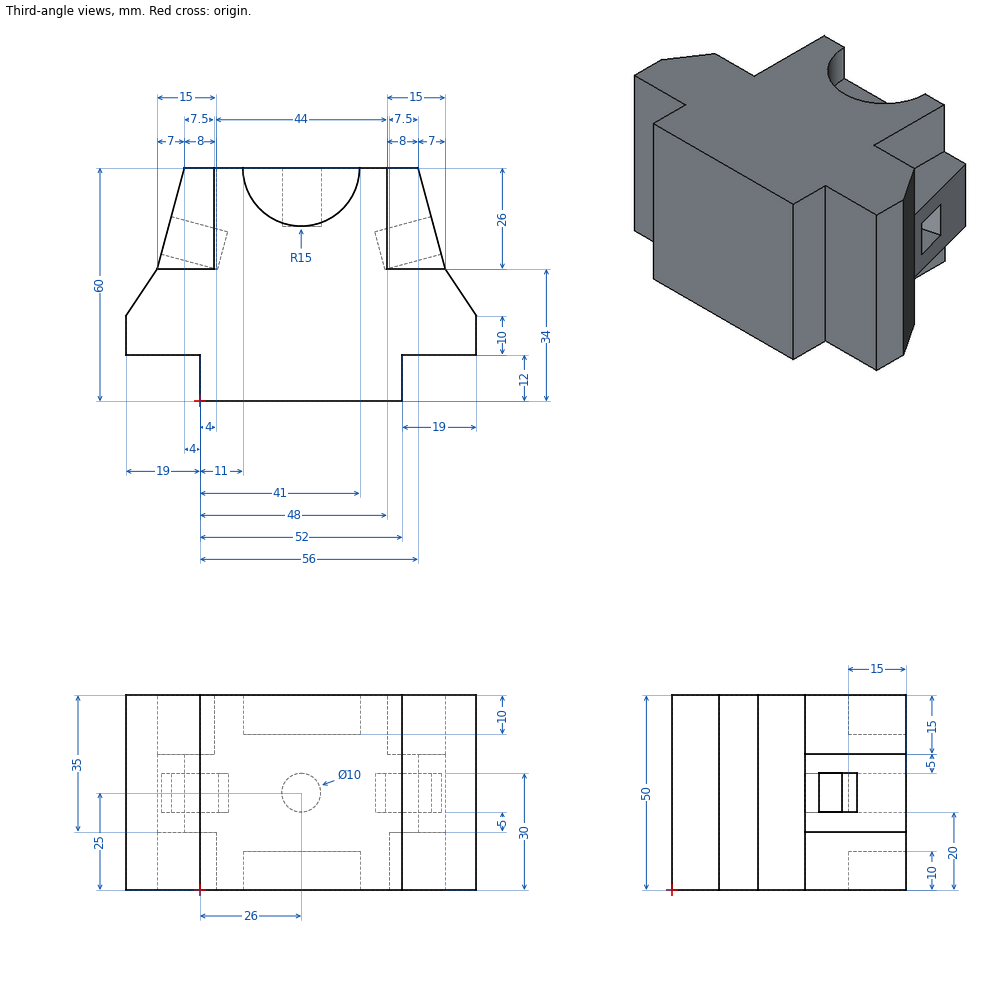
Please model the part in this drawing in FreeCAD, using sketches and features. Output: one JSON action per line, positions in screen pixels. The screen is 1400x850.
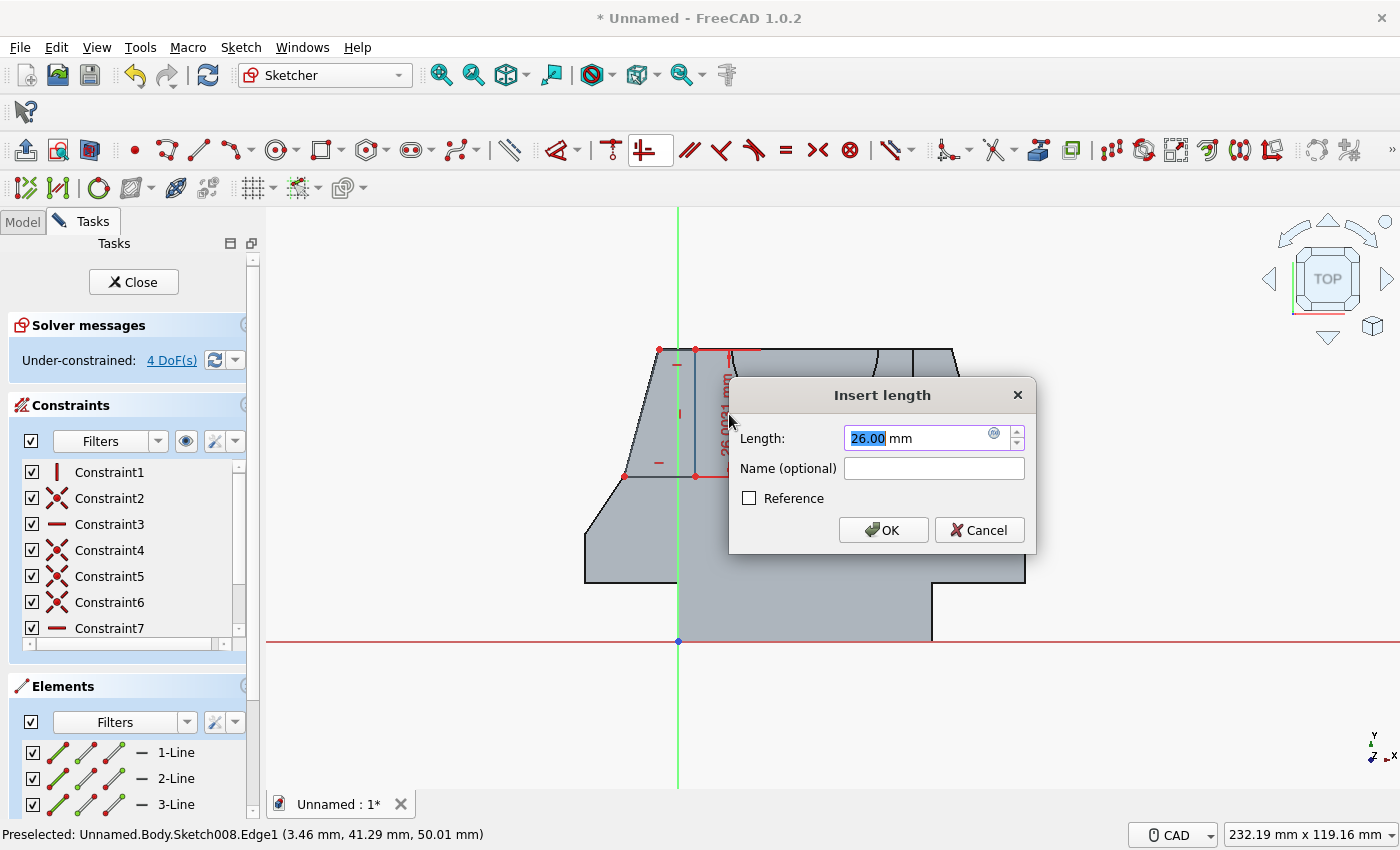
{"action": "type", "text": "26"}
{"action": "key", "text": "Return"}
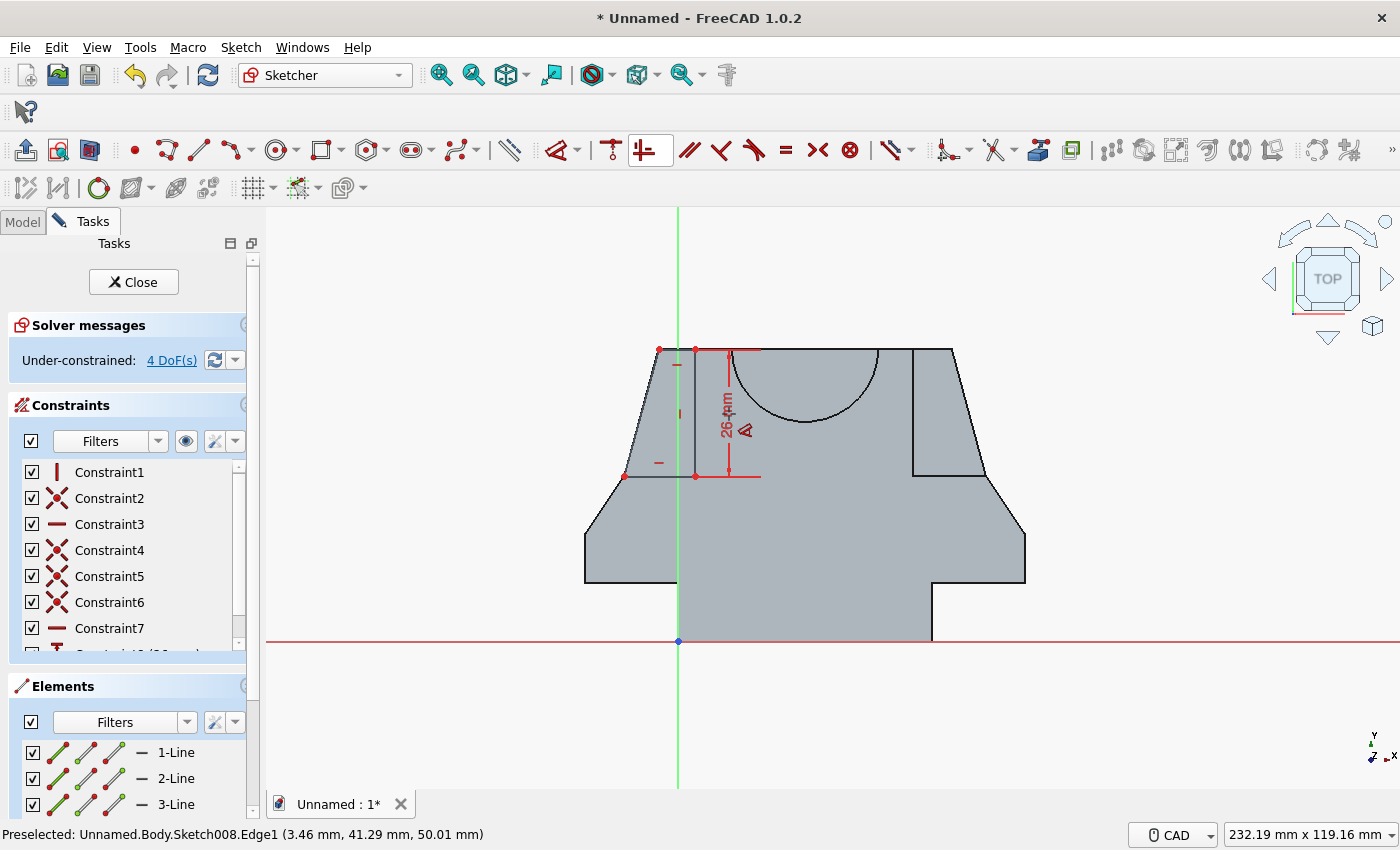
{"action": "scroll", "coordinate": [659, 350], "scroll_direction": "up", "scroll_amount": 4}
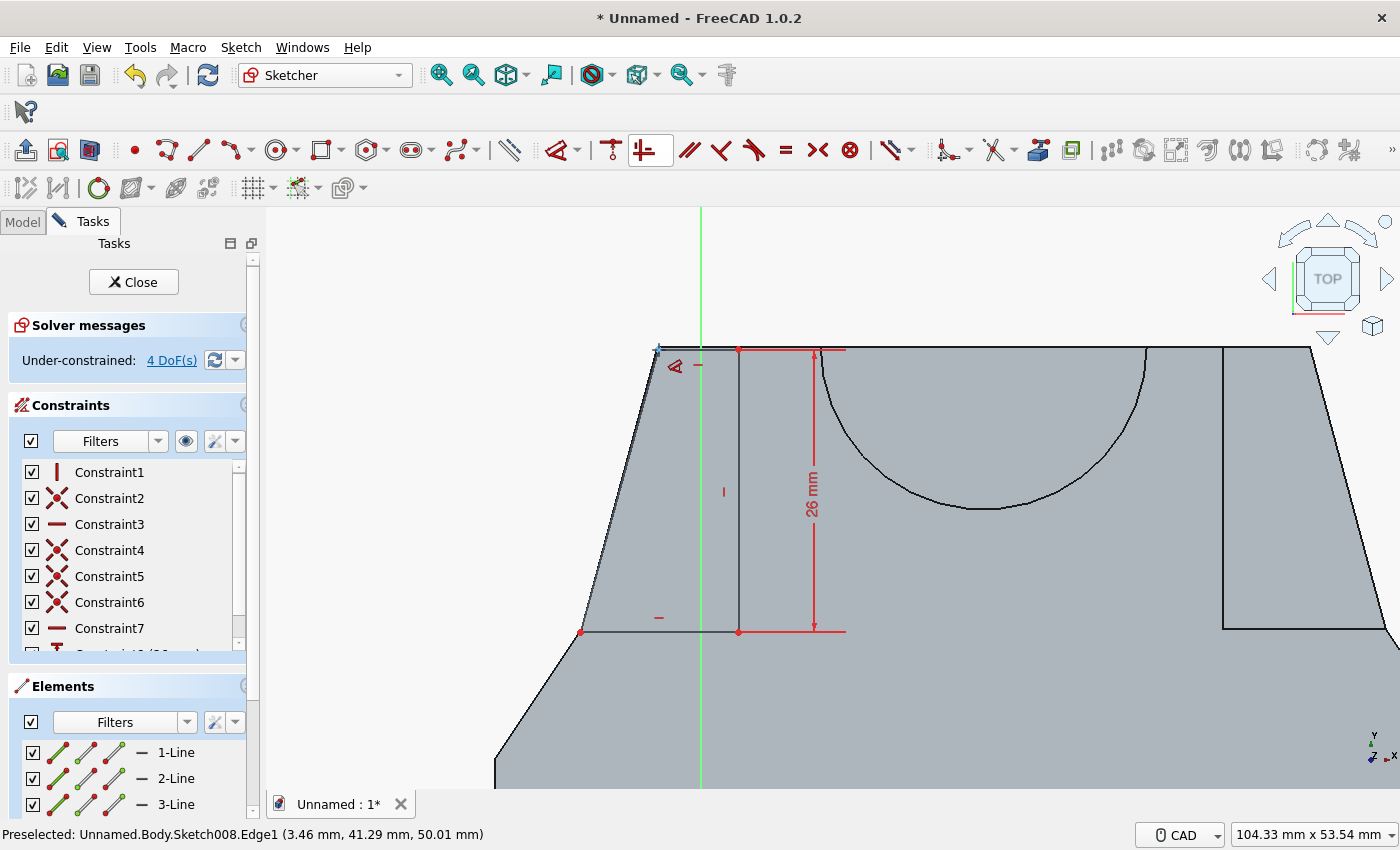
{"action": "left_click", "coordinate": [659, 350]}
{"action": "left_click", "coordinate": [680, 316]}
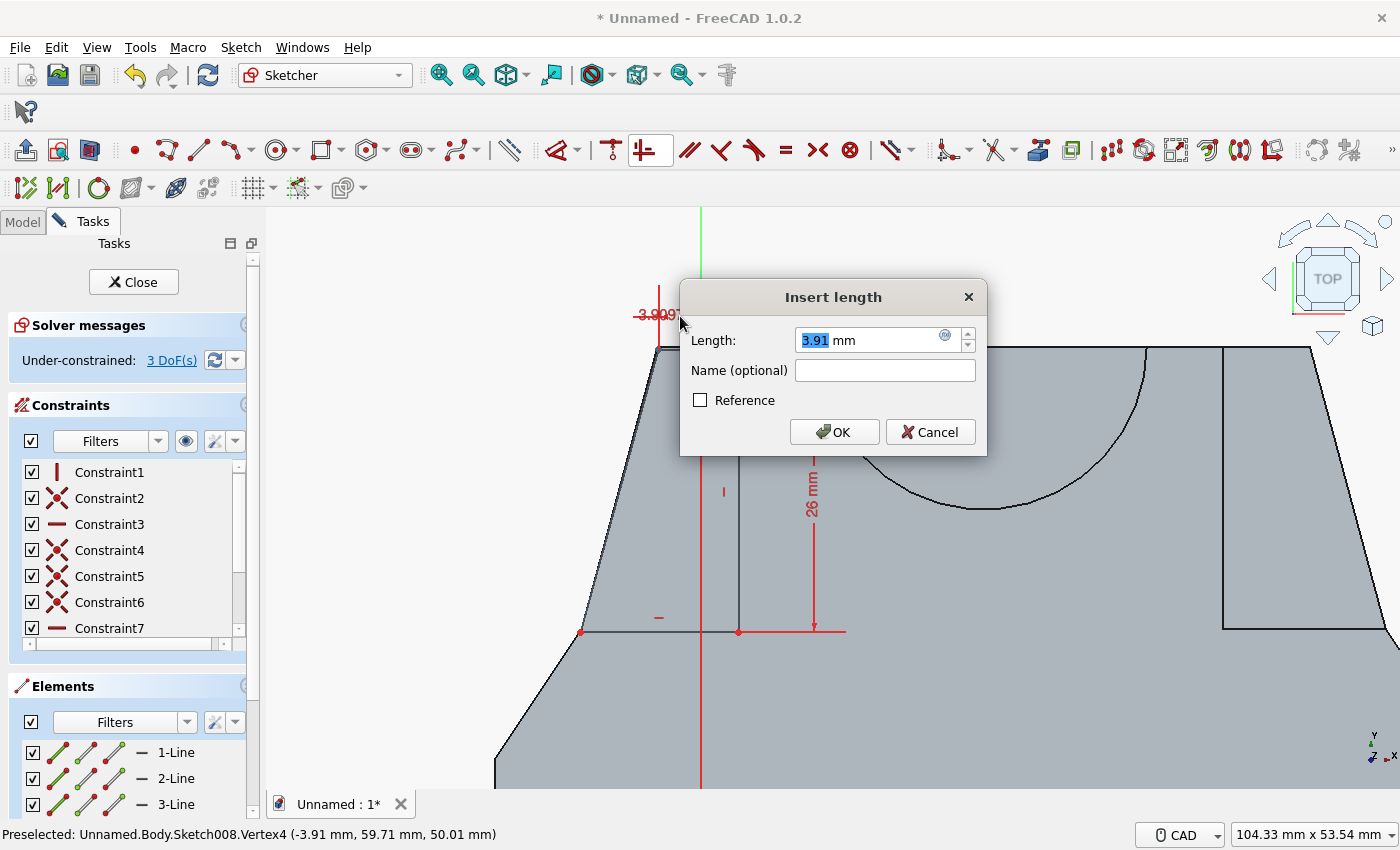
{"action": "type", "text": "4"}
{"action": "key", "text": "Return"}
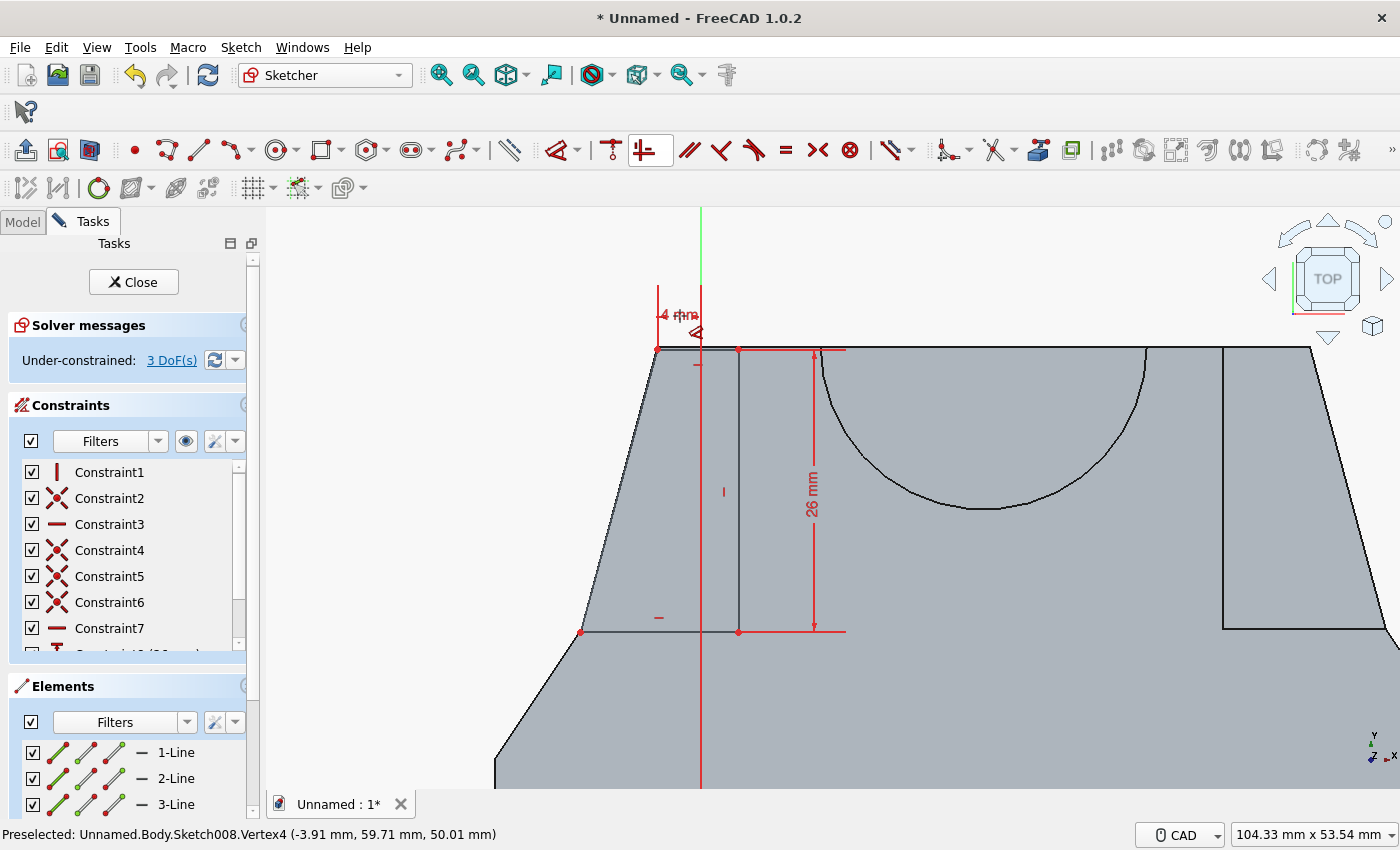
{"action": "left_click", "coordinate": [635, 434]}
{"action": "left_click", "coordinate": [601, 316]}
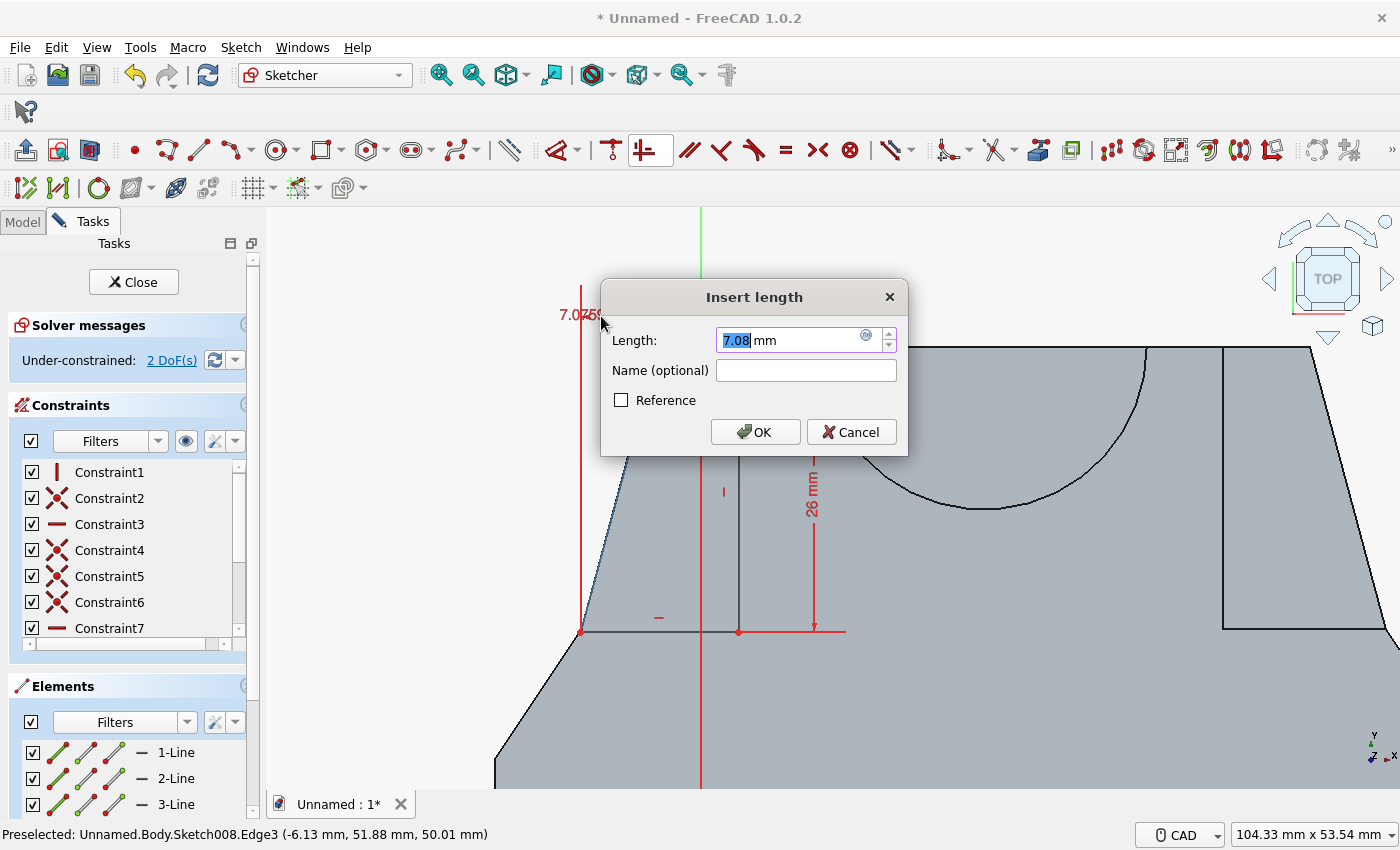
{"action": "type", "text": "7"}
{"action": "key", "text": "Return"}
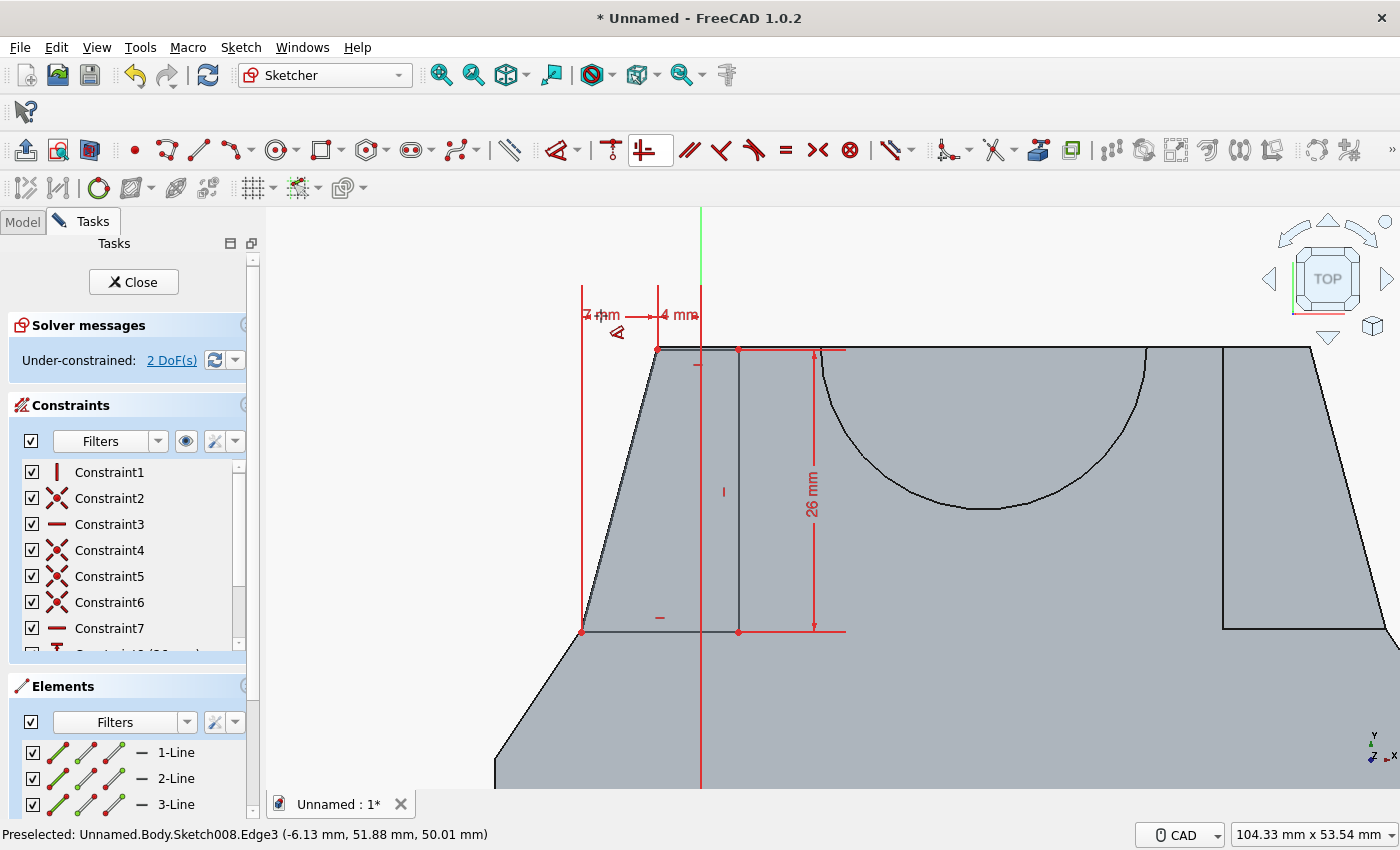
{"action": "left_click", "coordinate": [714, 350]}
{"action": "left_click", "coordinate": [679, 384]}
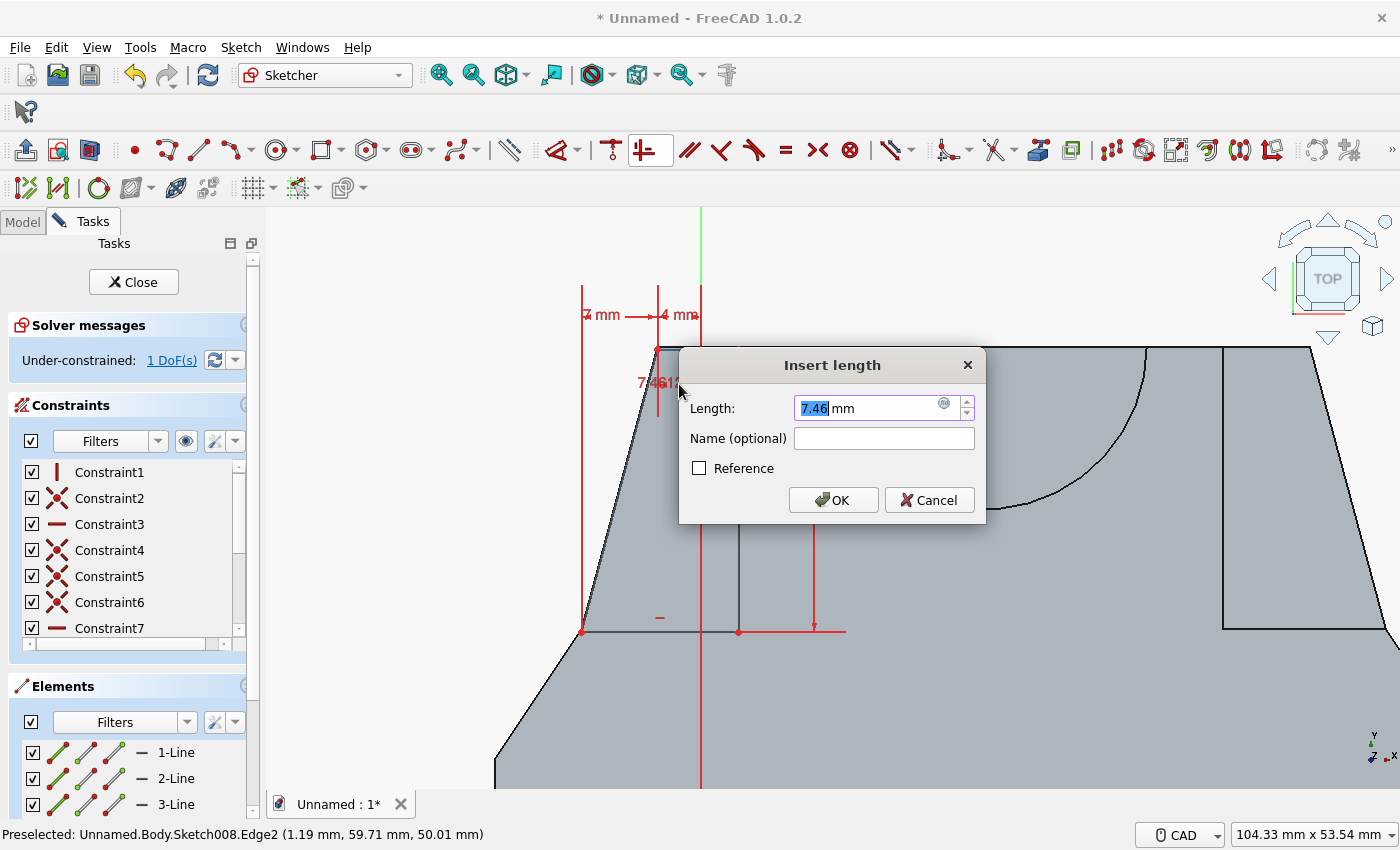
{"action": "type", "text": "7.5"}
{"action": "key", "text": "Return"}